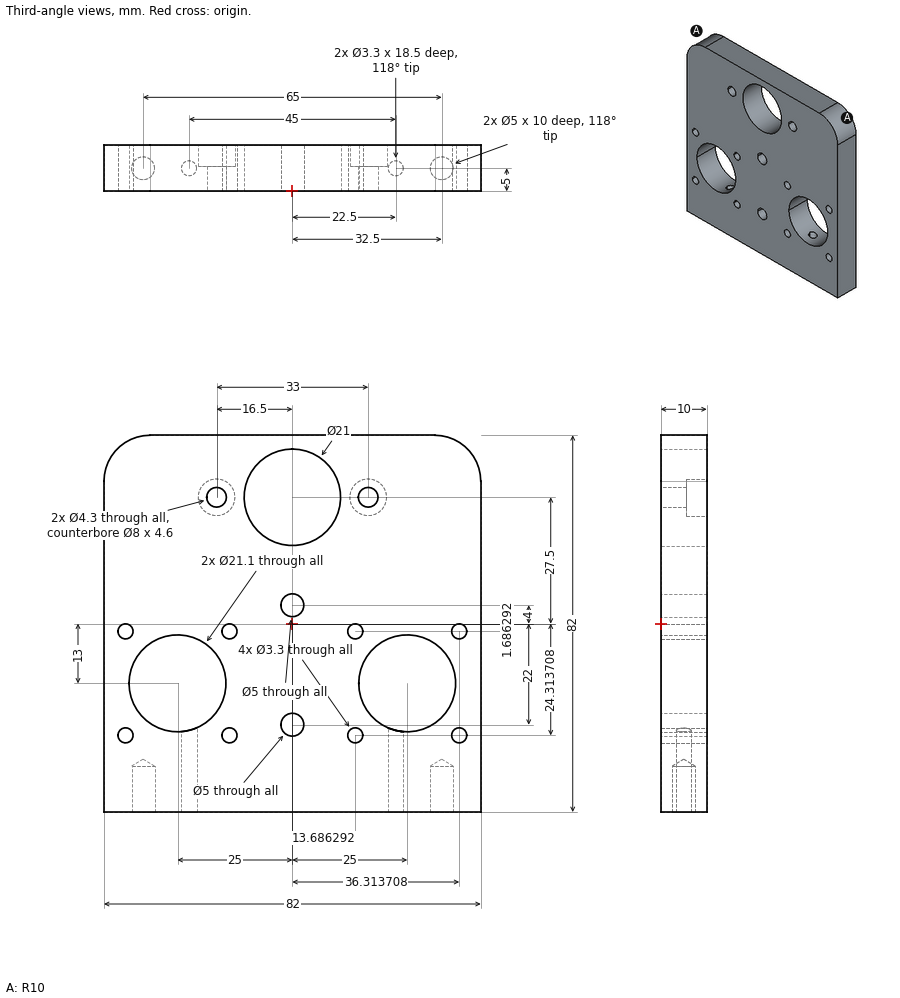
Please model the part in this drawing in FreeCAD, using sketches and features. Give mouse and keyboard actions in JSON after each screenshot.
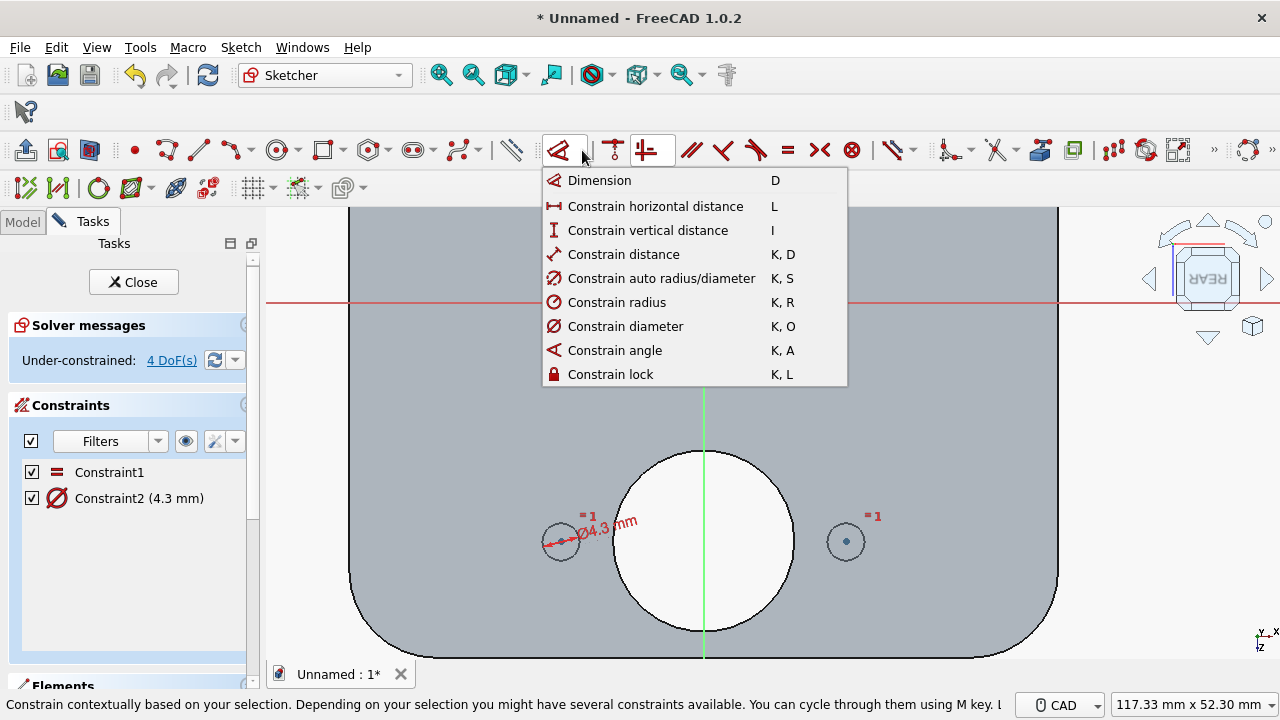
{"action": "left_click", "coordinate": [695, 206]}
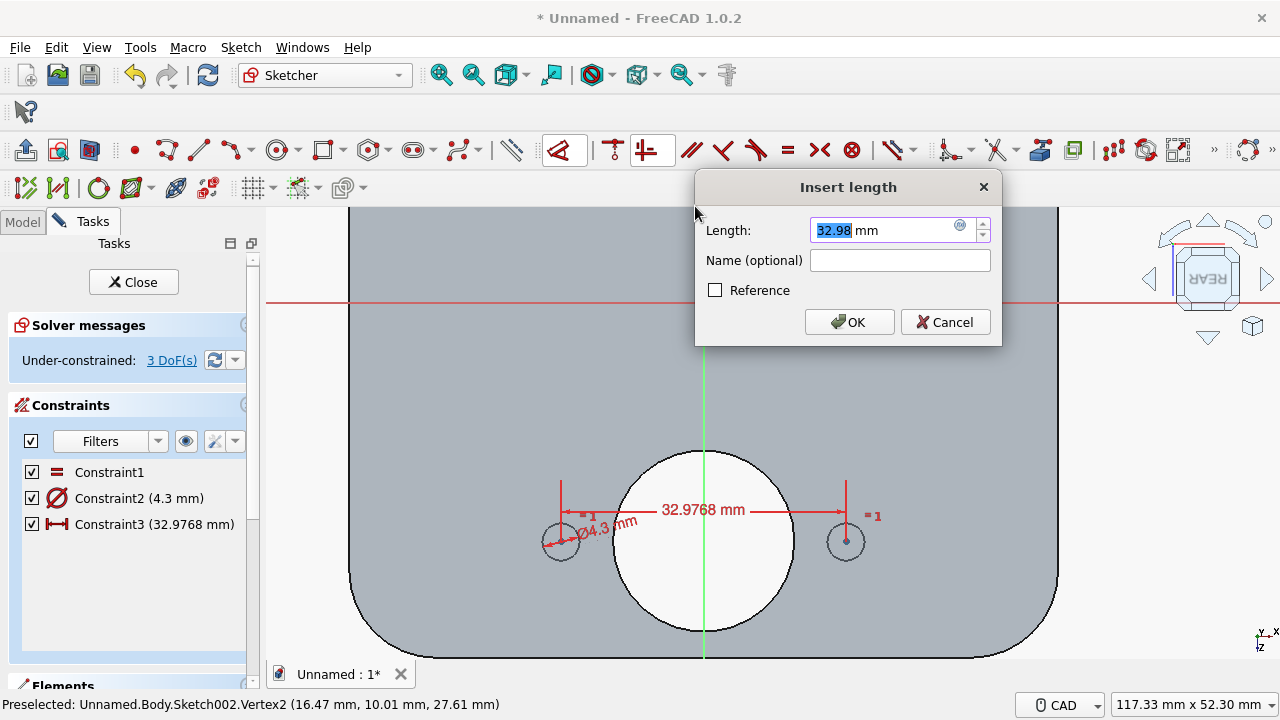
{"action": "type", "text": "33"}
{"action": "key", "text": "Return"}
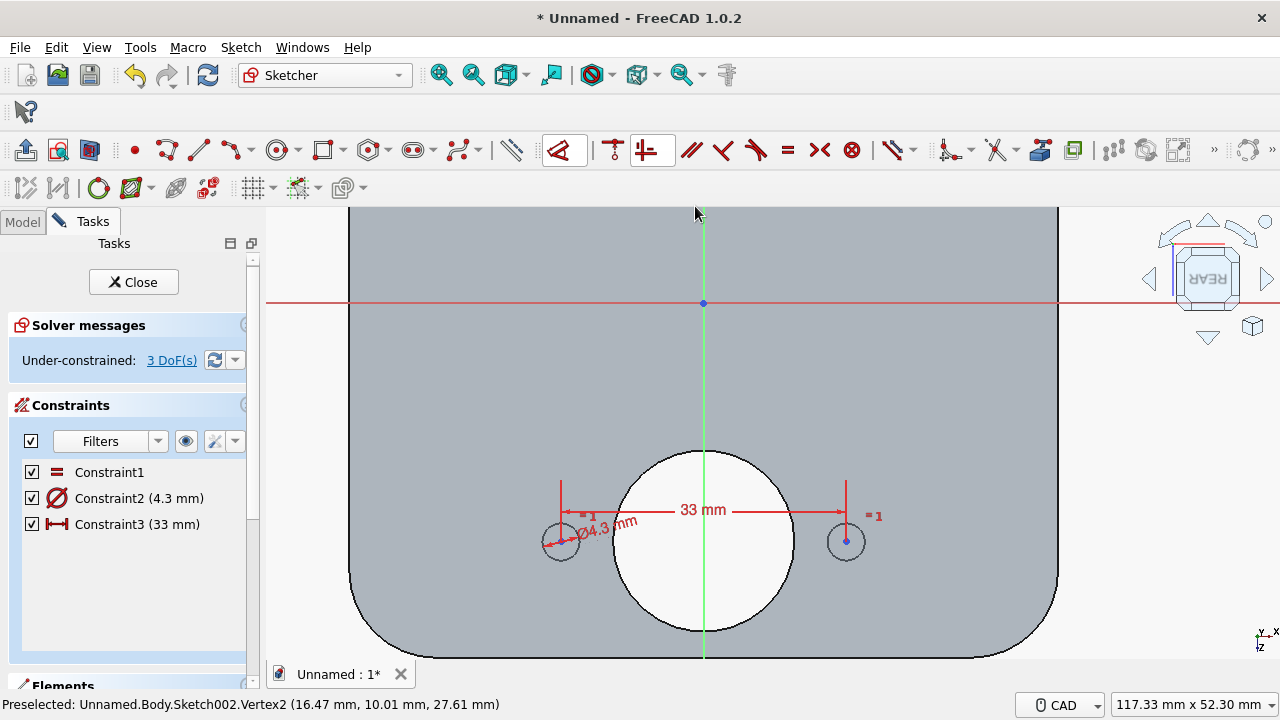
{"action": "left_click", "coordinate": [561, 542]}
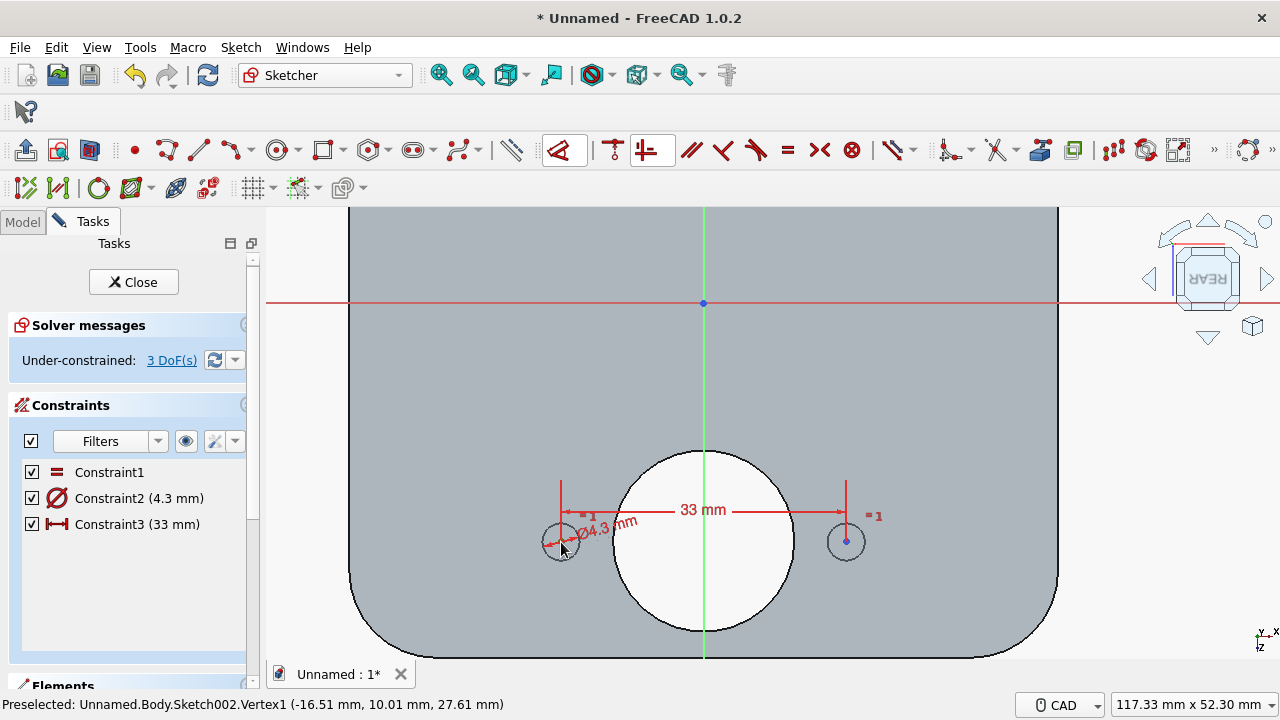
{"action": "left_click", "coordinate": [582, 150]}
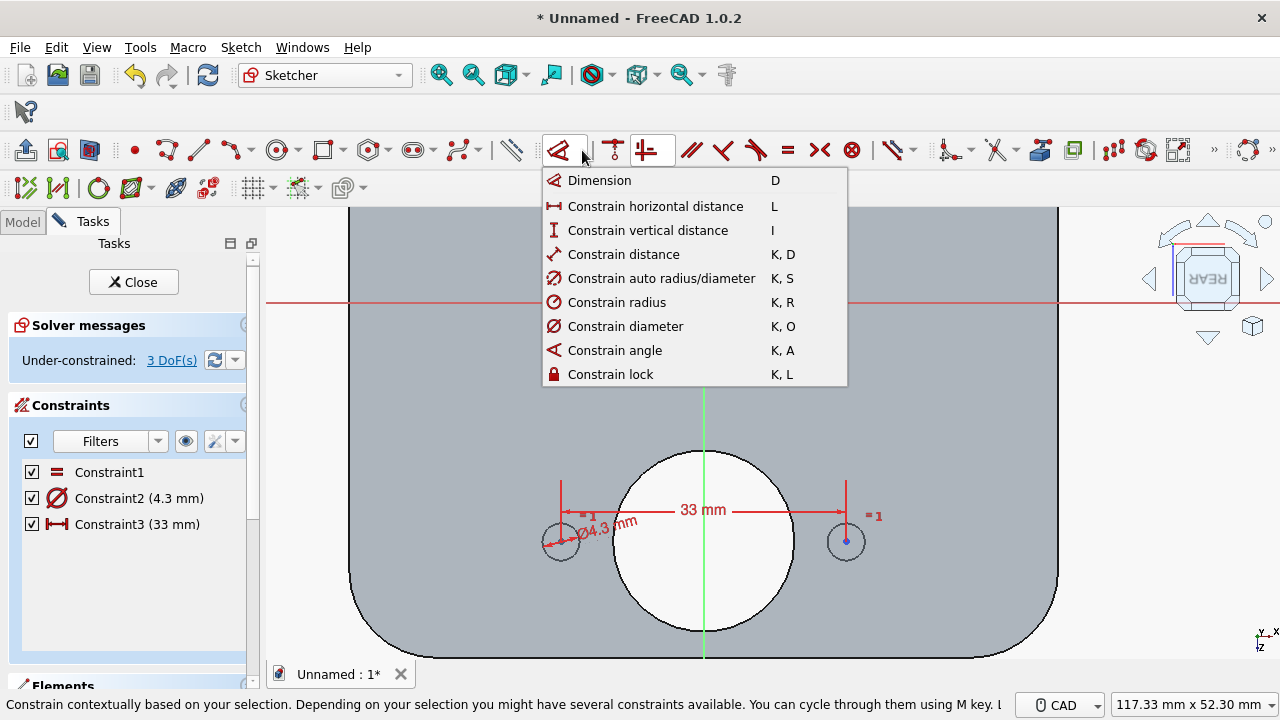
{"action": "left_click", "coordinate": [695, 206]}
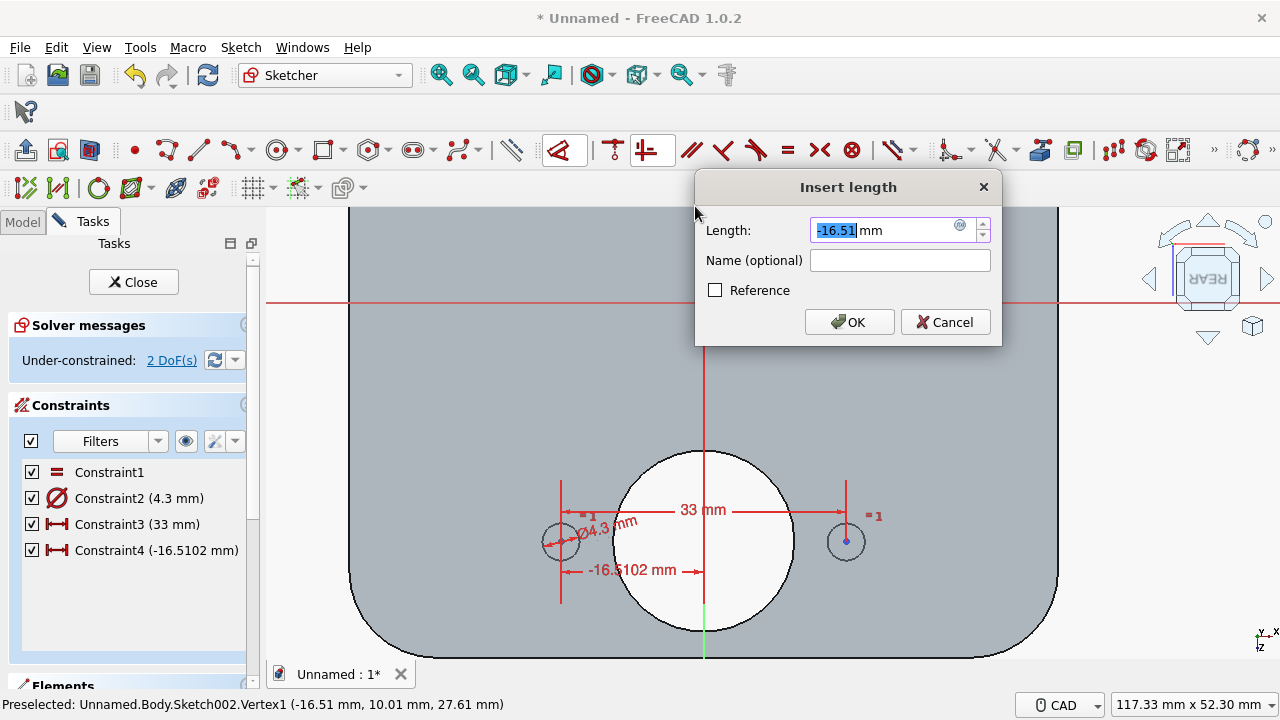
{"action": "type", "text": "-16.5"}
{"action": "key", "text": "Return"}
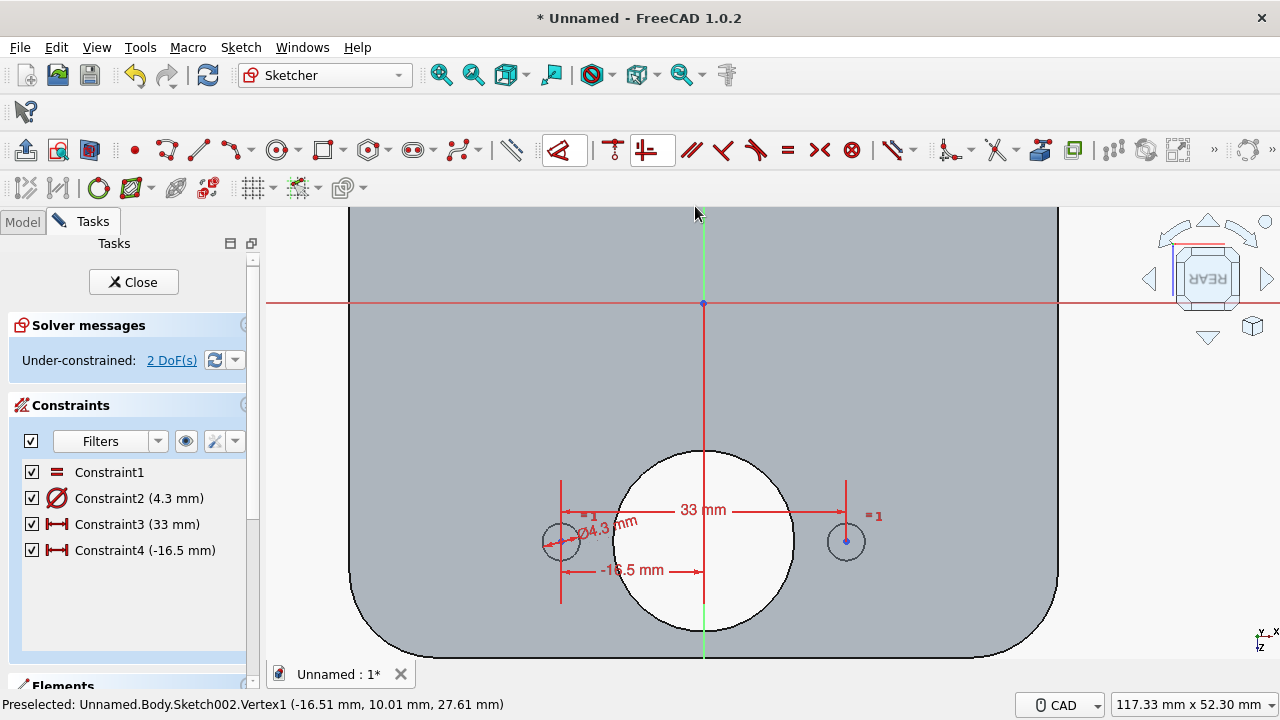
{"action": "left_click", "coordinate": [561, 542]}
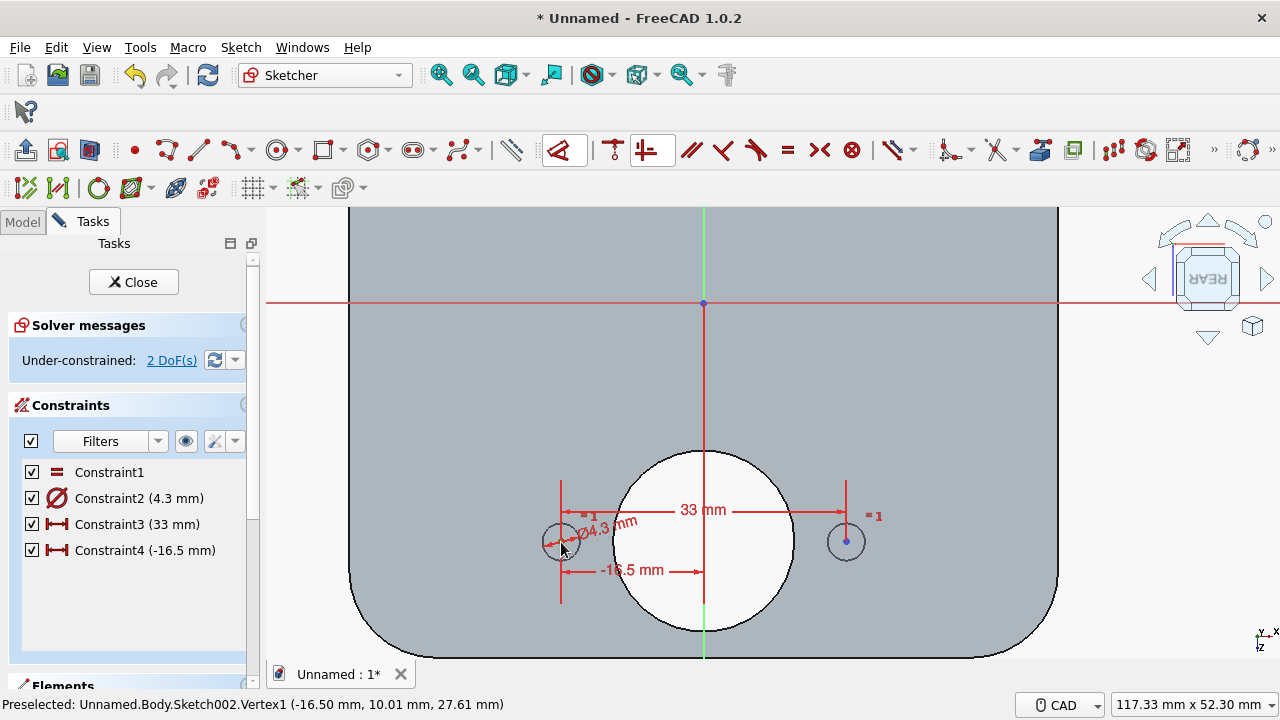
{"action": "key", "text": "i"}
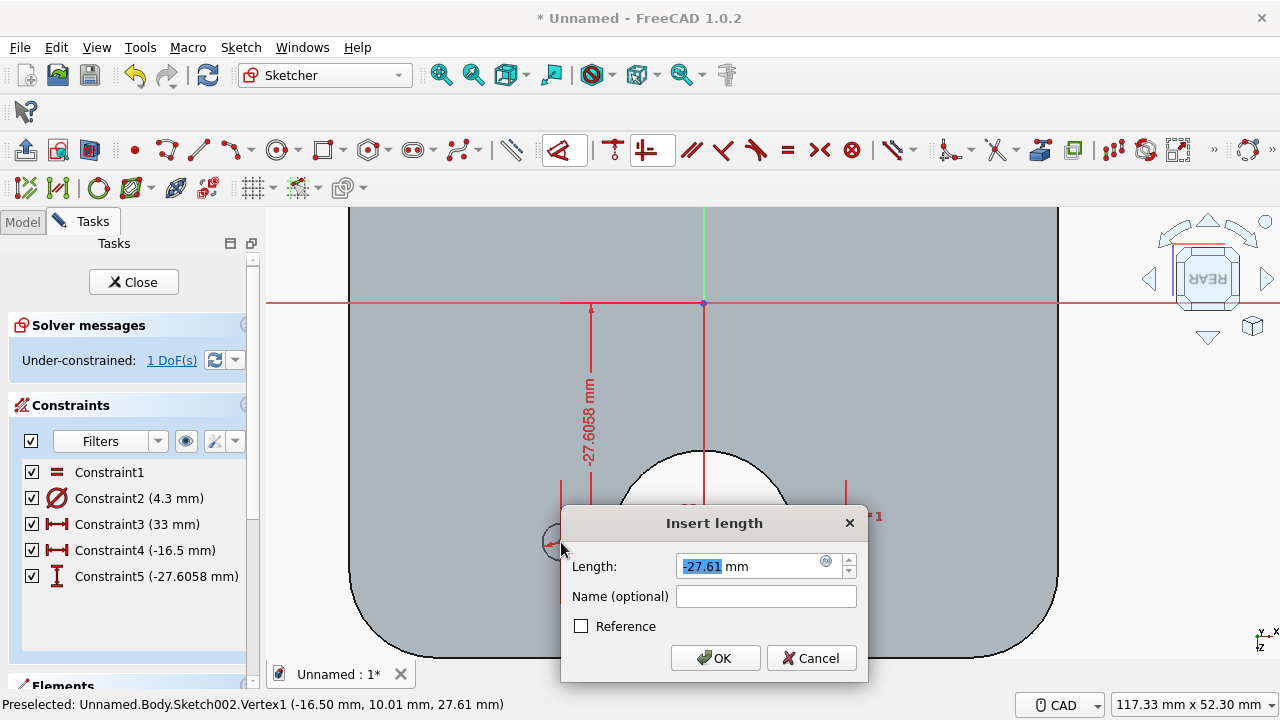
{"action": "type", "text": "-27.5"}
{"action": "key", "text": "Return"}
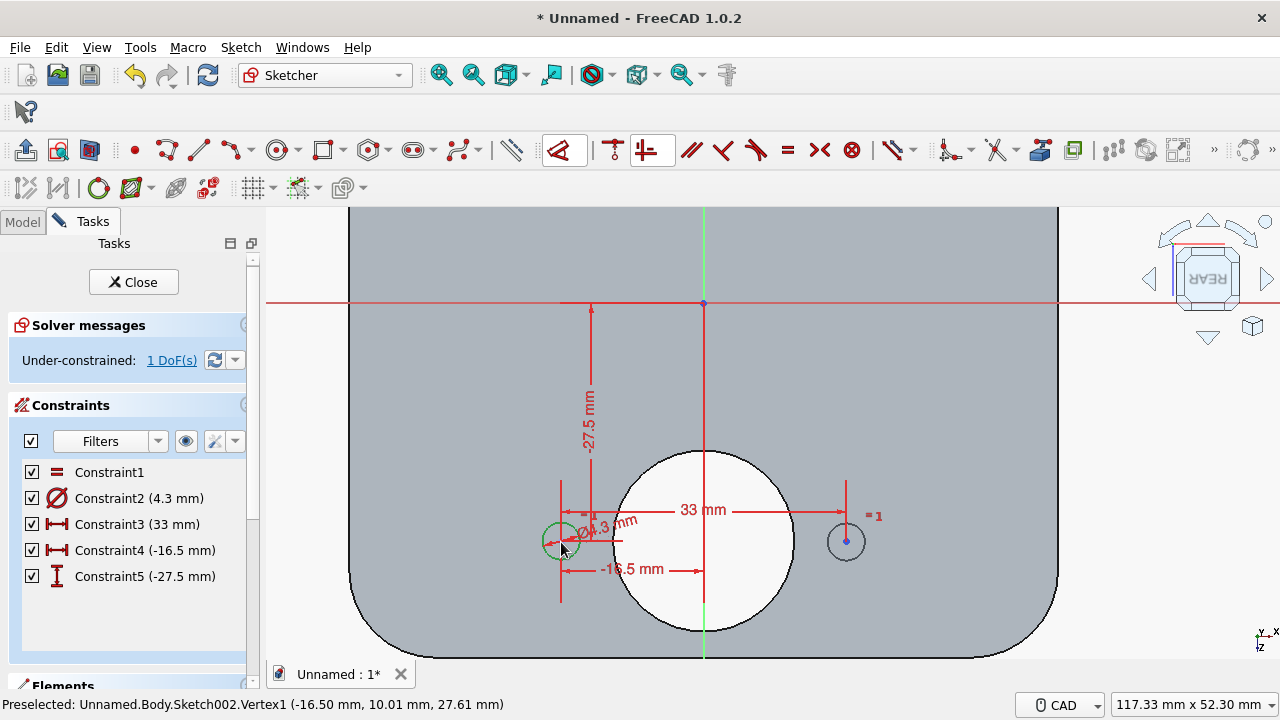
{"action": "left_click", "coordinate": [846, 542]}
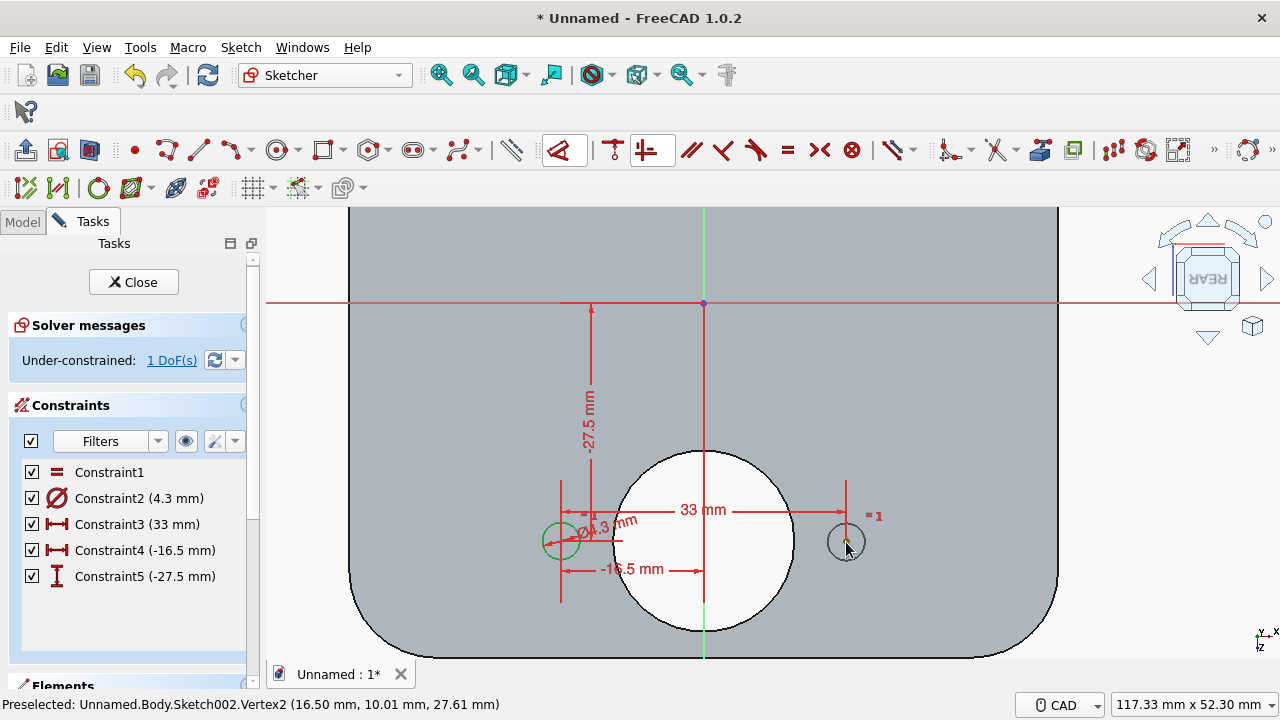
{"action": "left_click", "coordinate": [582, 150]}